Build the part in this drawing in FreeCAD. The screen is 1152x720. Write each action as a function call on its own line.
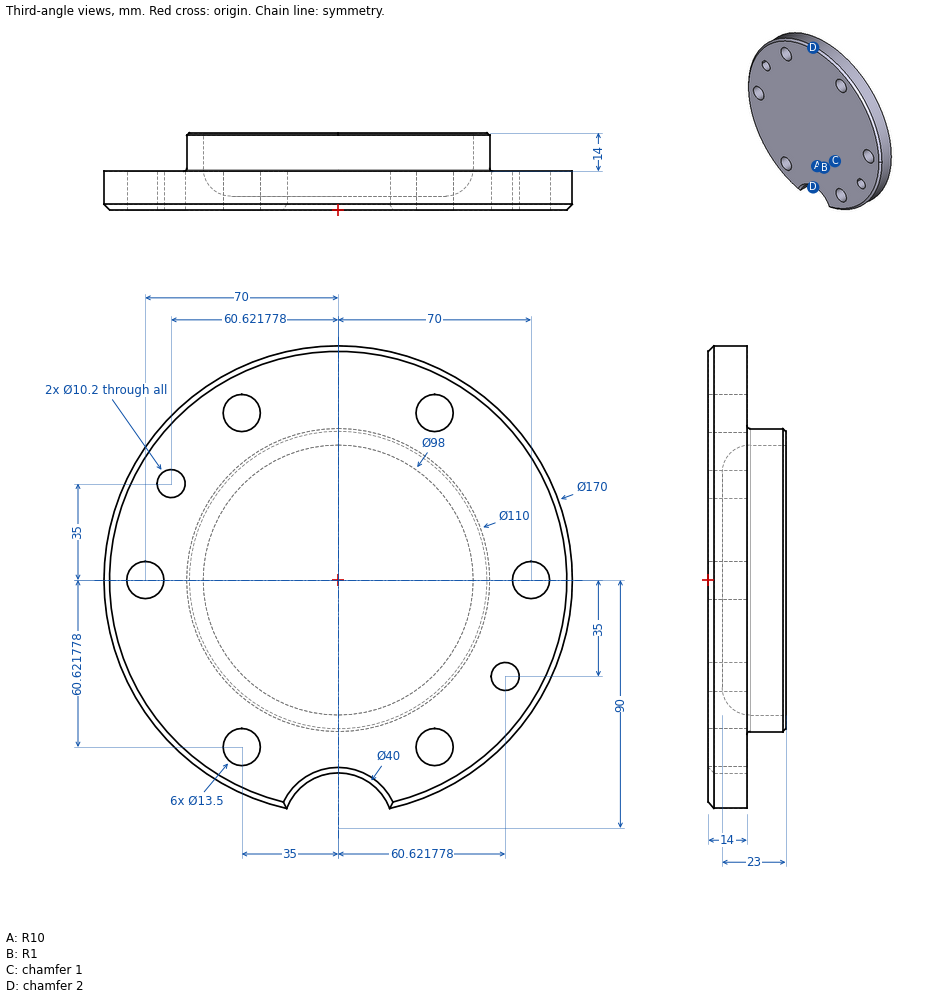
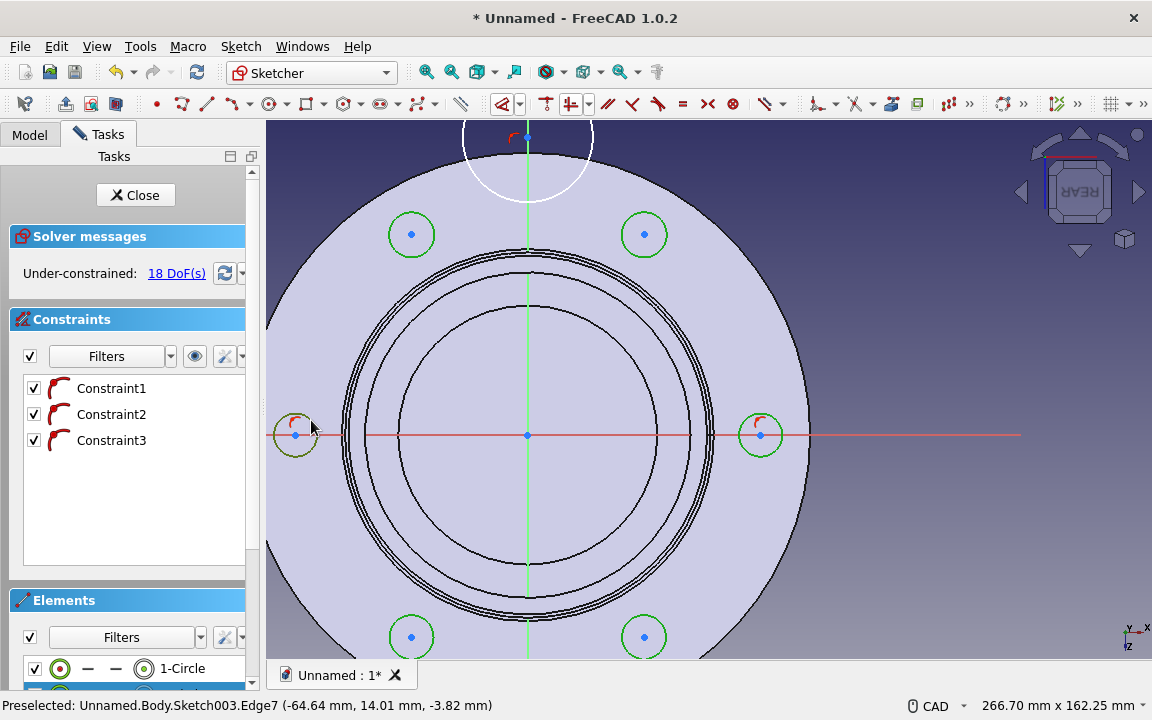
click(683, 104)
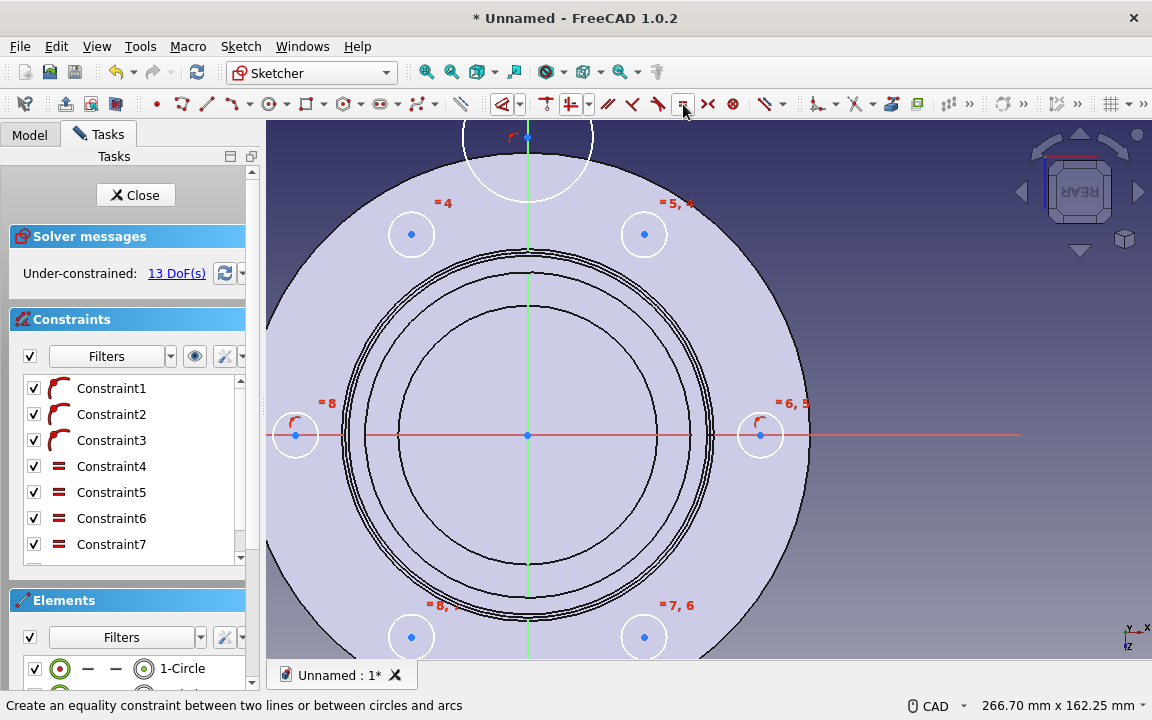
click(412, 235)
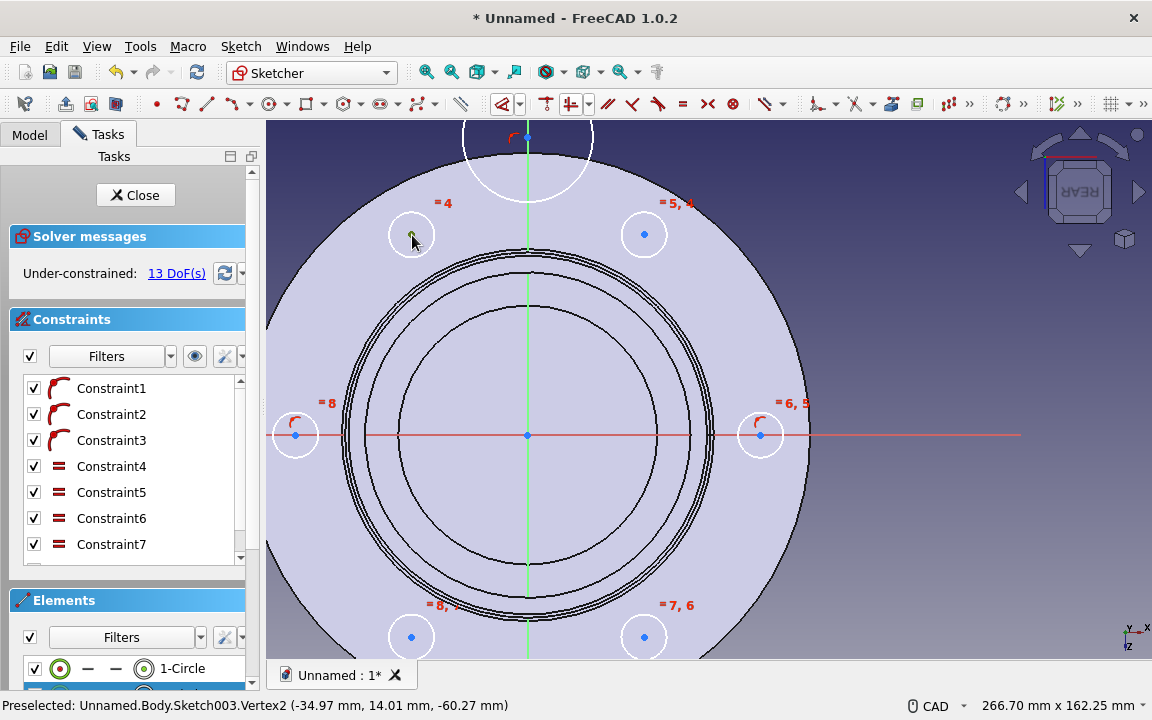
click(644, 235)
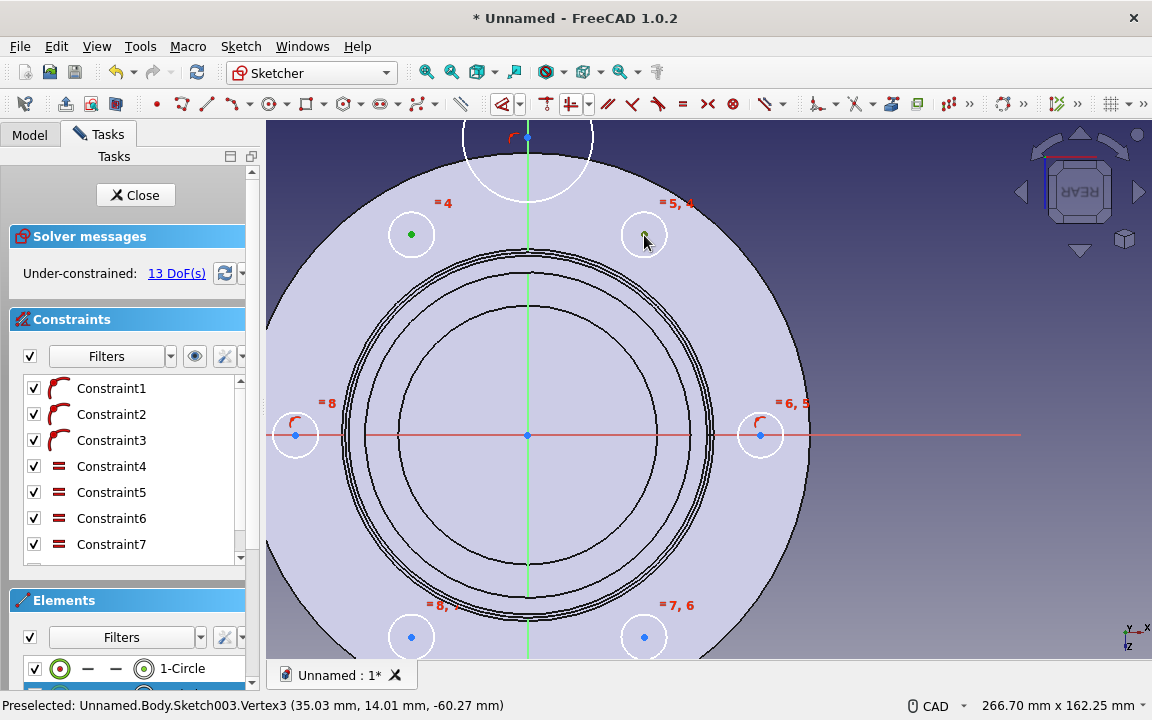
click(528, 596)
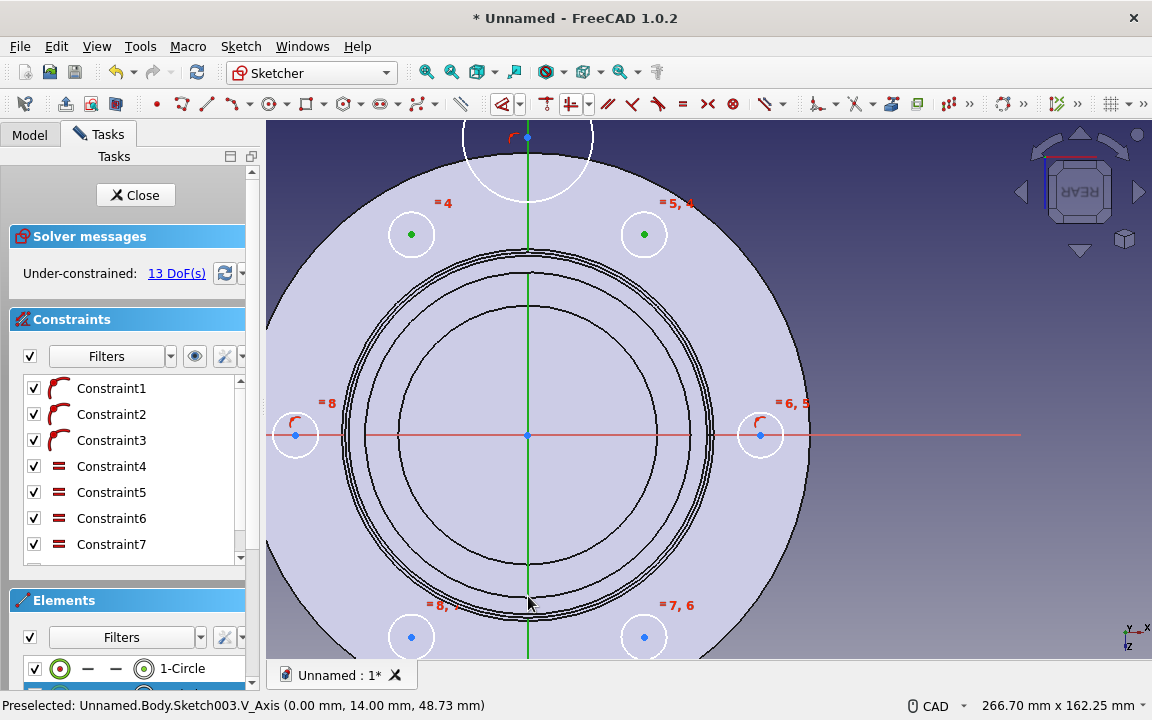
click(708, 104)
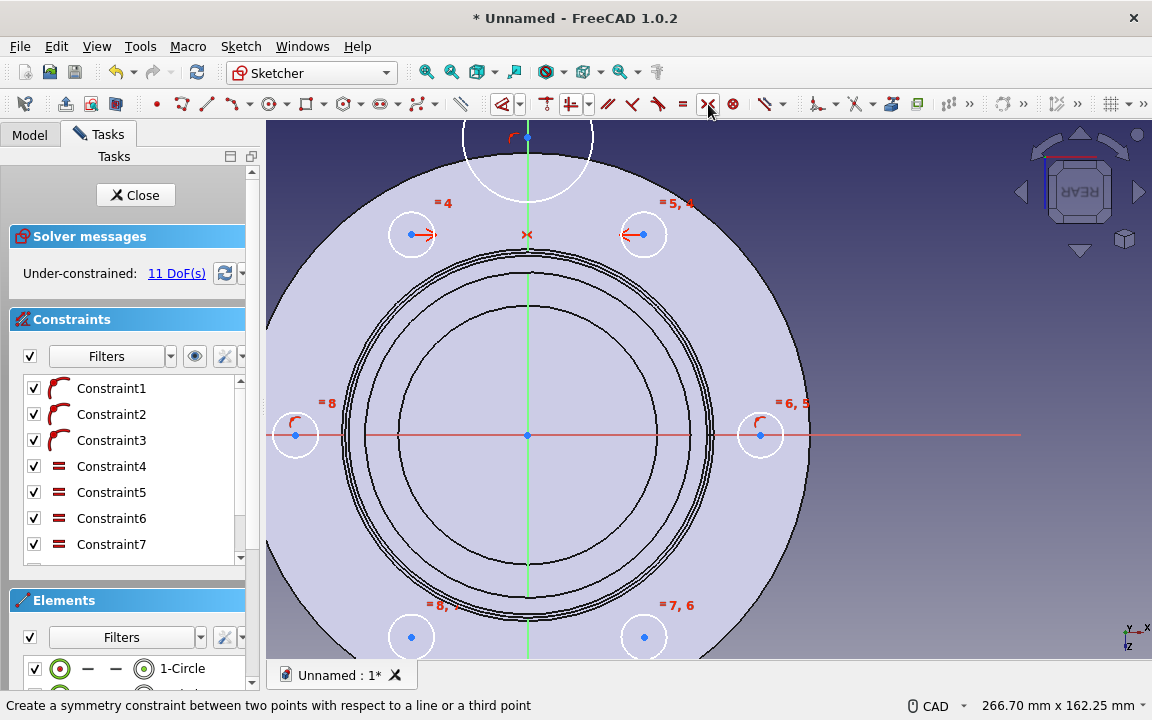
click(644, 235)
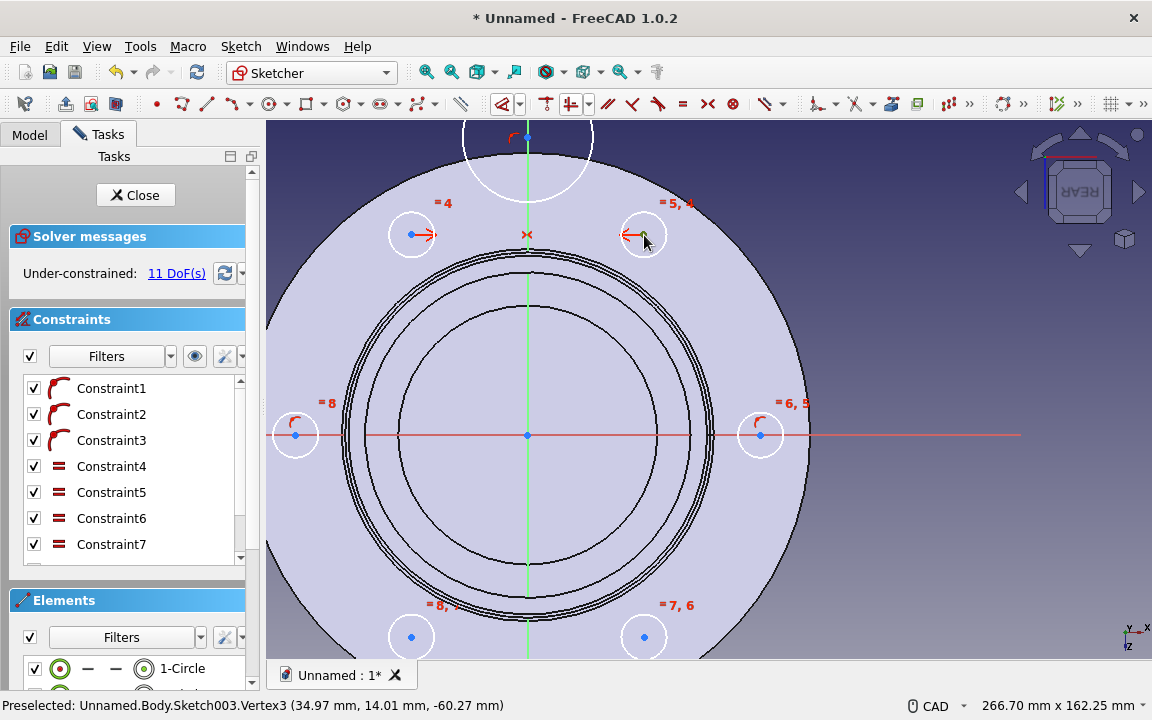
scroll(778, 420, down, 3)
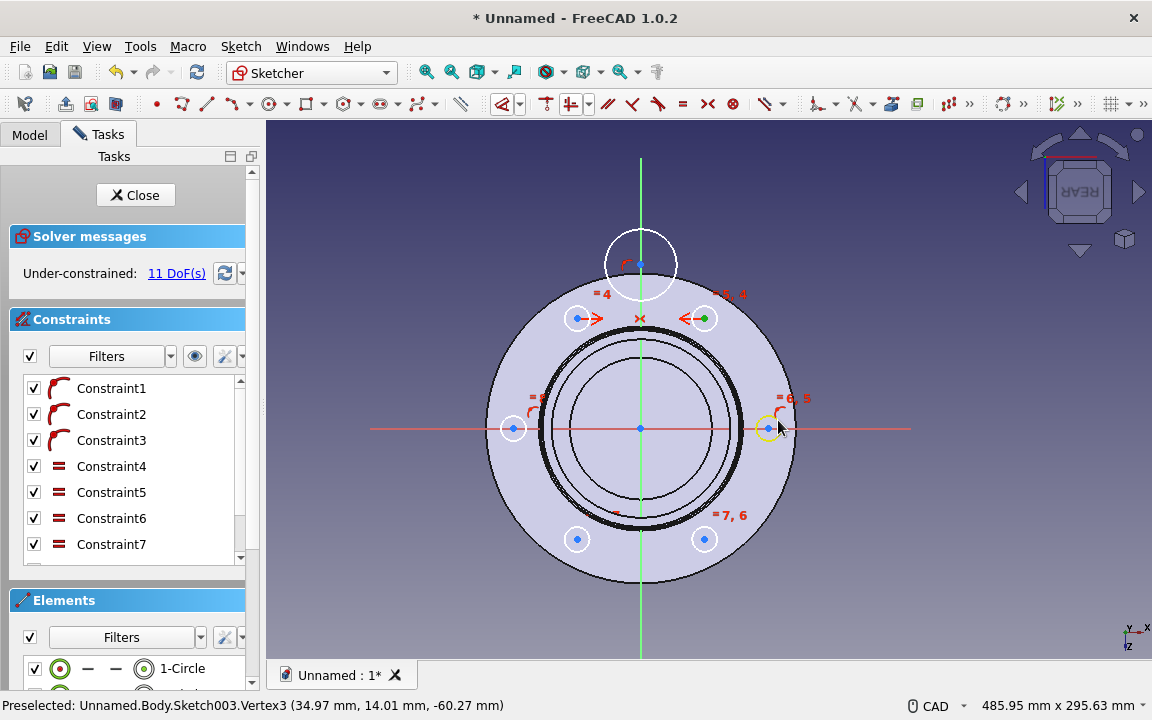
click(705, 539)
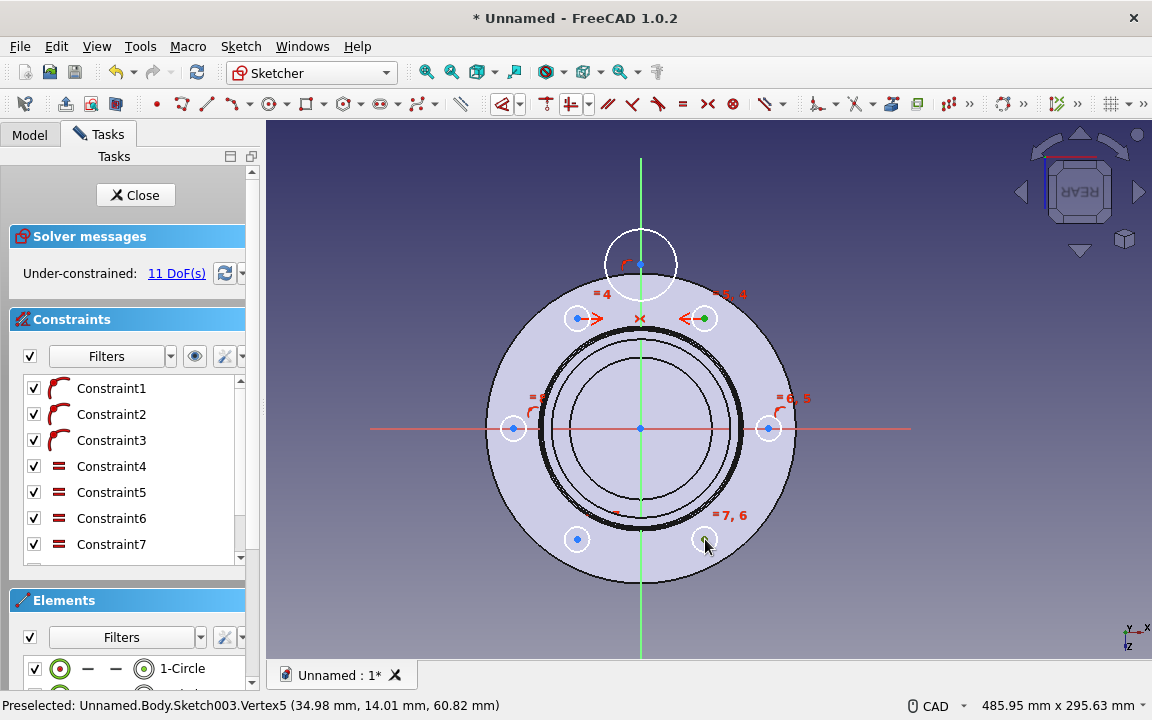
click(393, 429)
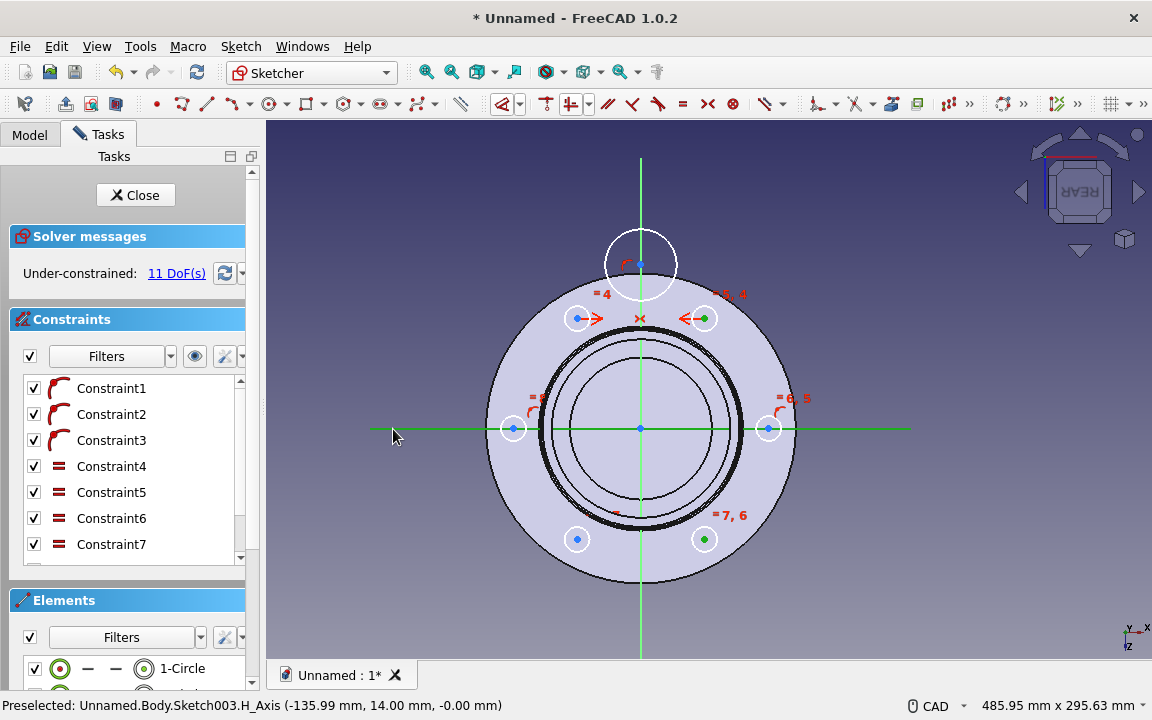
click(708, 104)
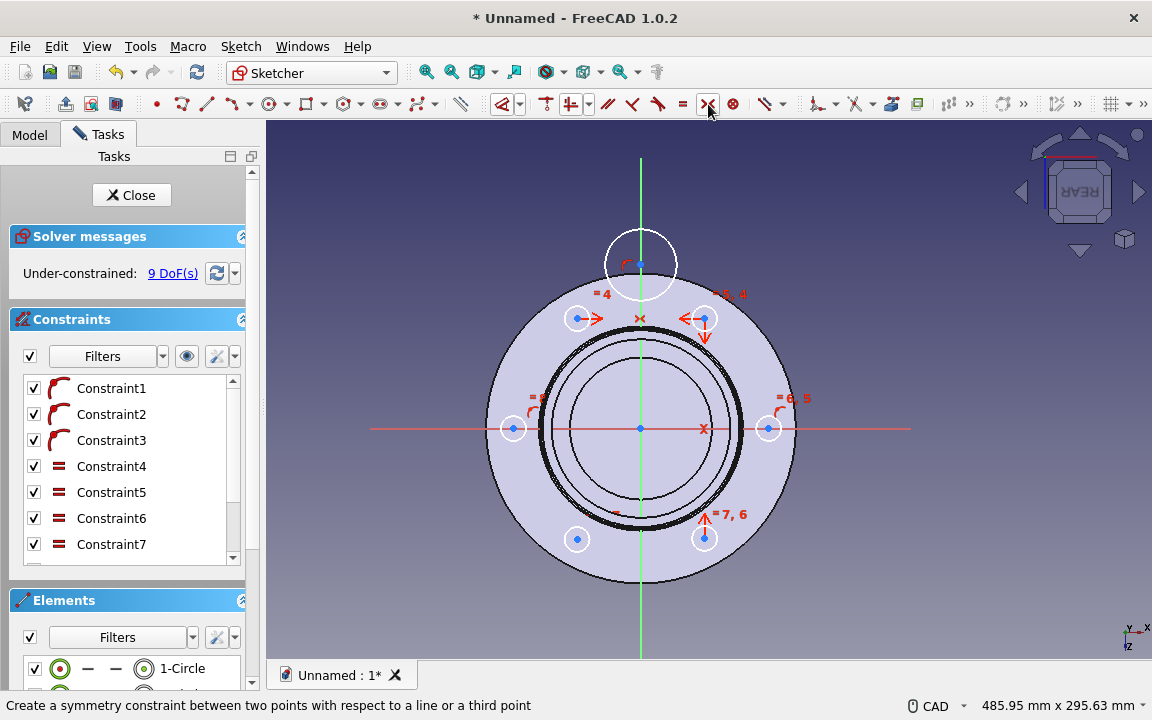
click(577, 319)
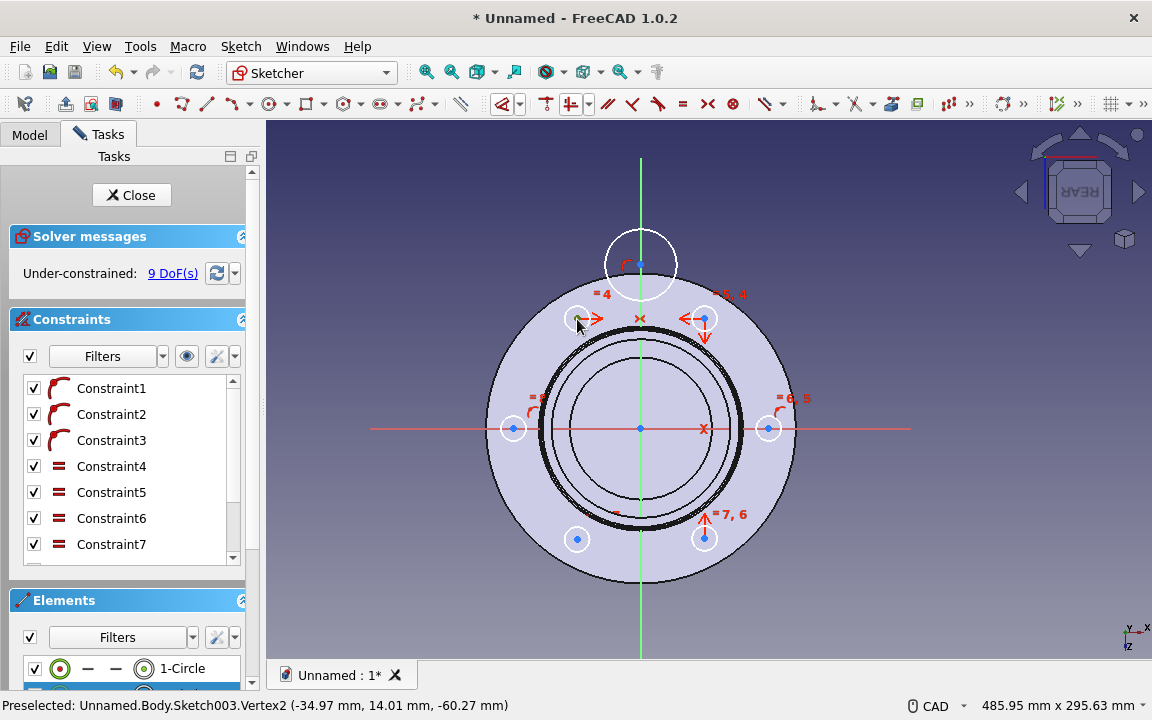
click(577, 539)